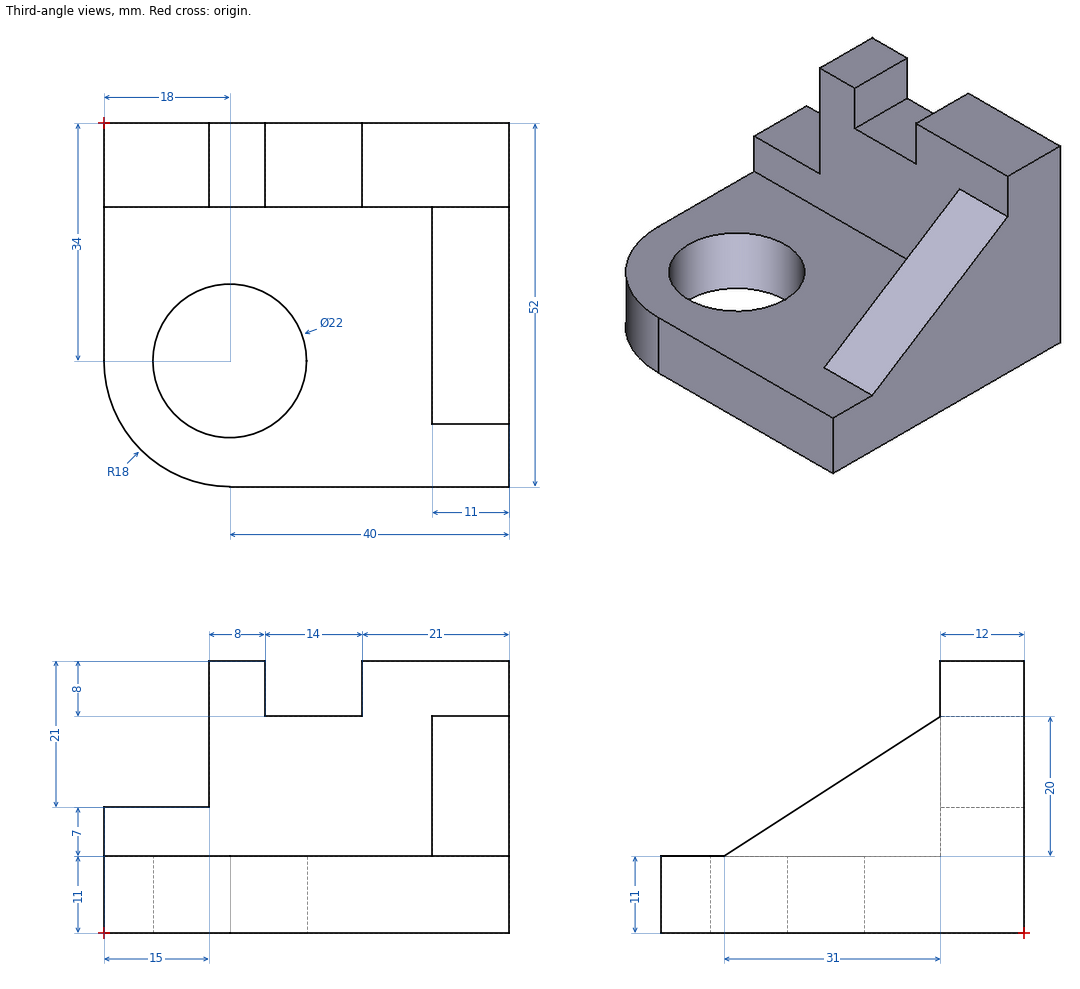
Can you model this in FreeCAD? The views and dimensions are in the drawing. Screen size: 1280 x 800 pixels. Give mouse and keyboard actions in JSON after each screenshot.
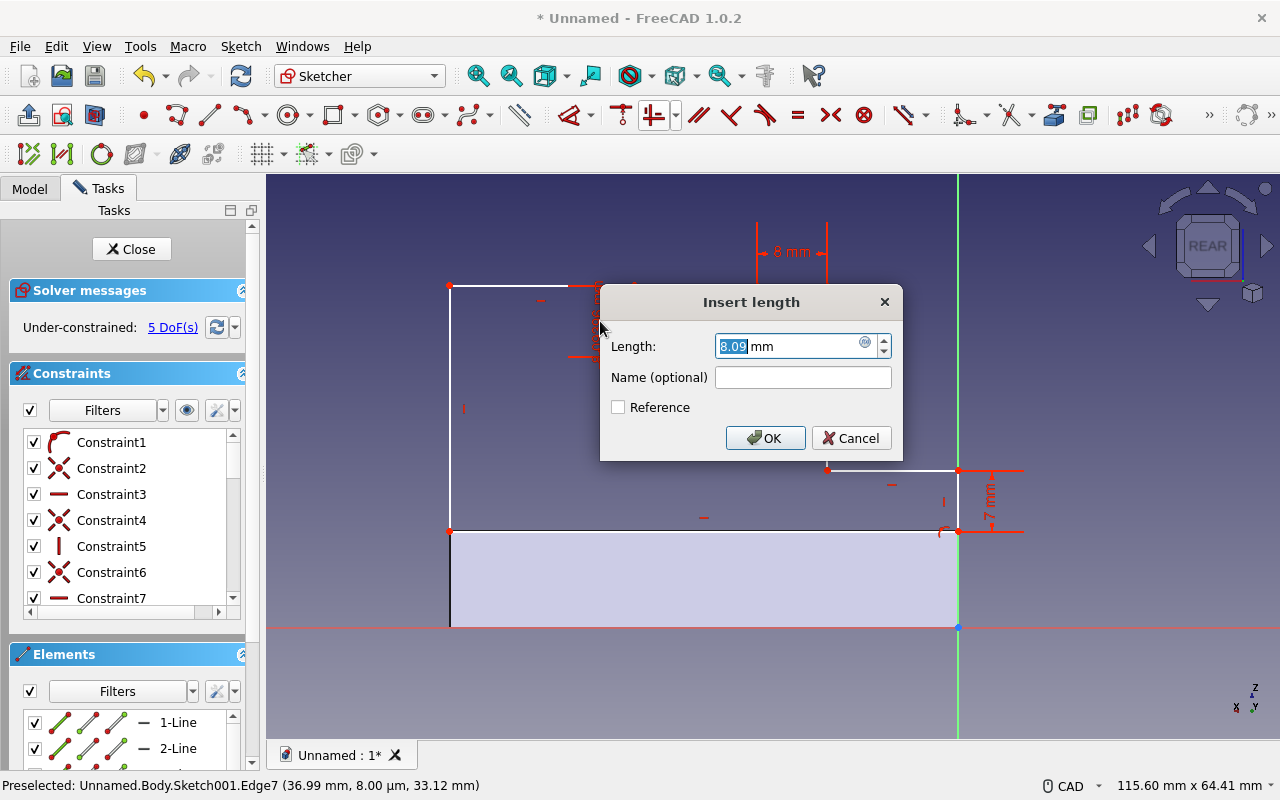
{"action": "type", "text": "8"}
{"action": "key", "text": "Return"}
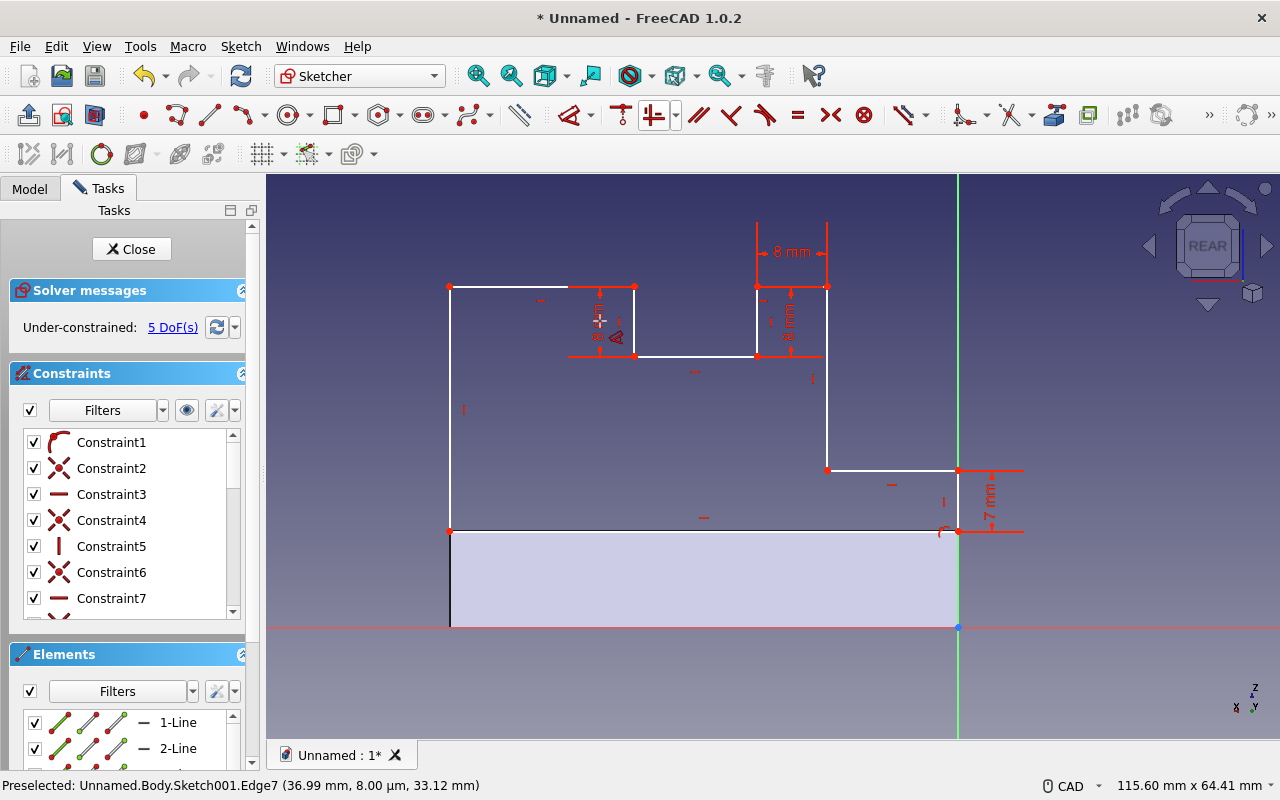
{"action": "left_click", "coordinate": [919, 471]}
{"action": "left_click", "coordinate": [893, 505]}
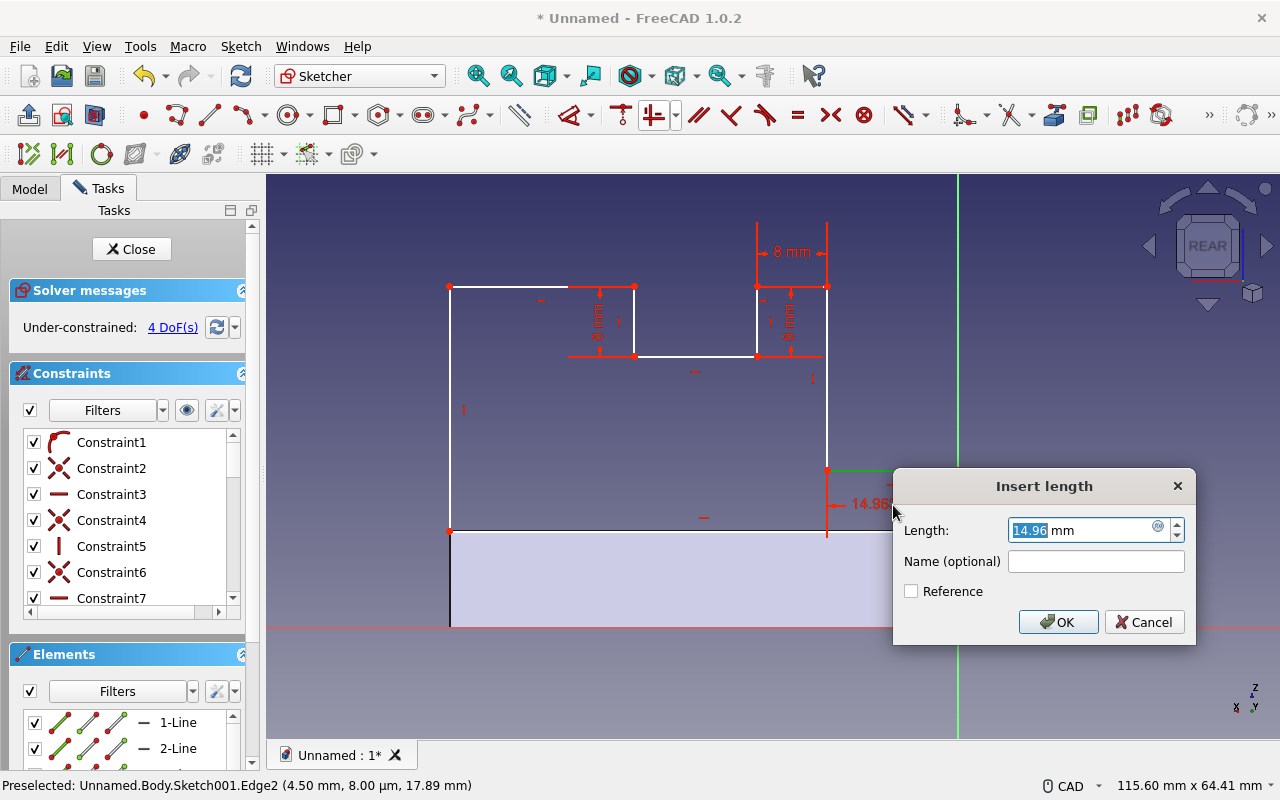
{"action": "type", "text": "15"}
{"action": "key", "text": "Return"}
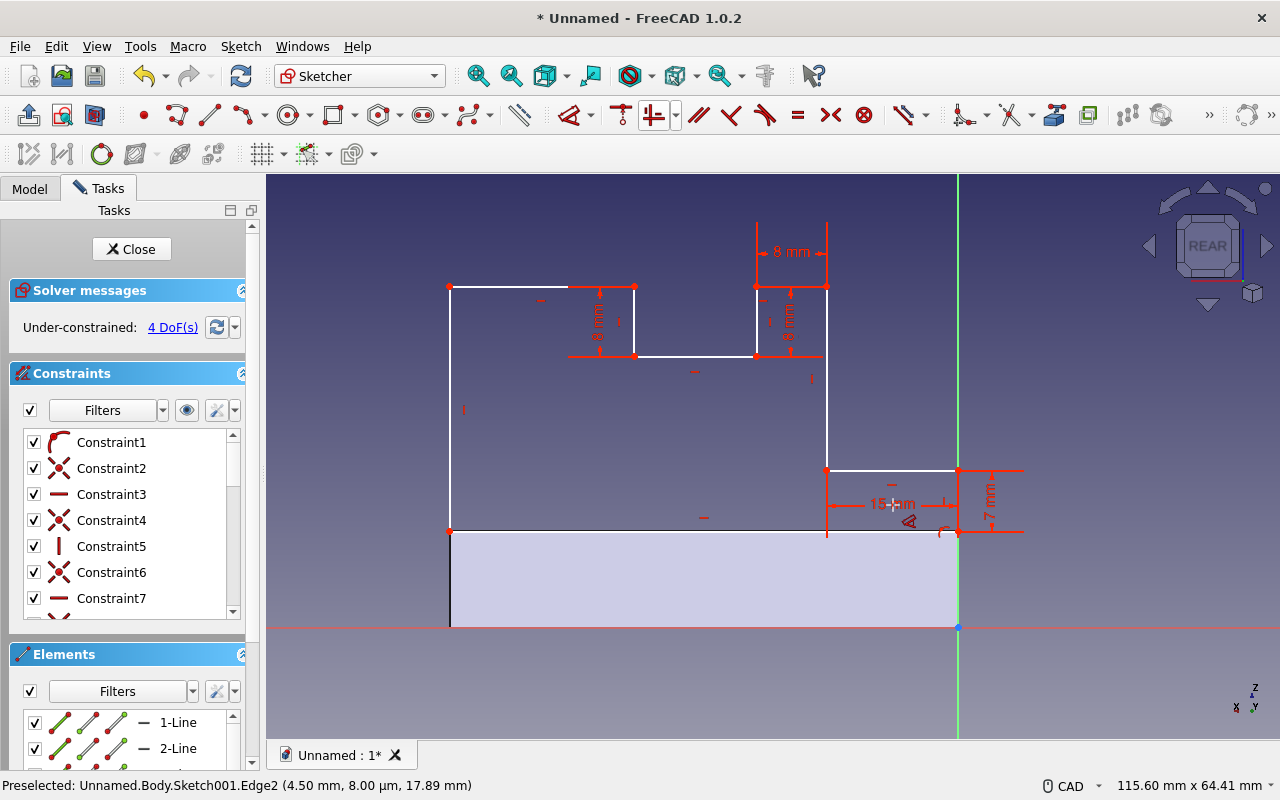
{"action": "left_click", "coordinate": [827, 415]}
{"action": "left_click", "coordinate": [861, 379]}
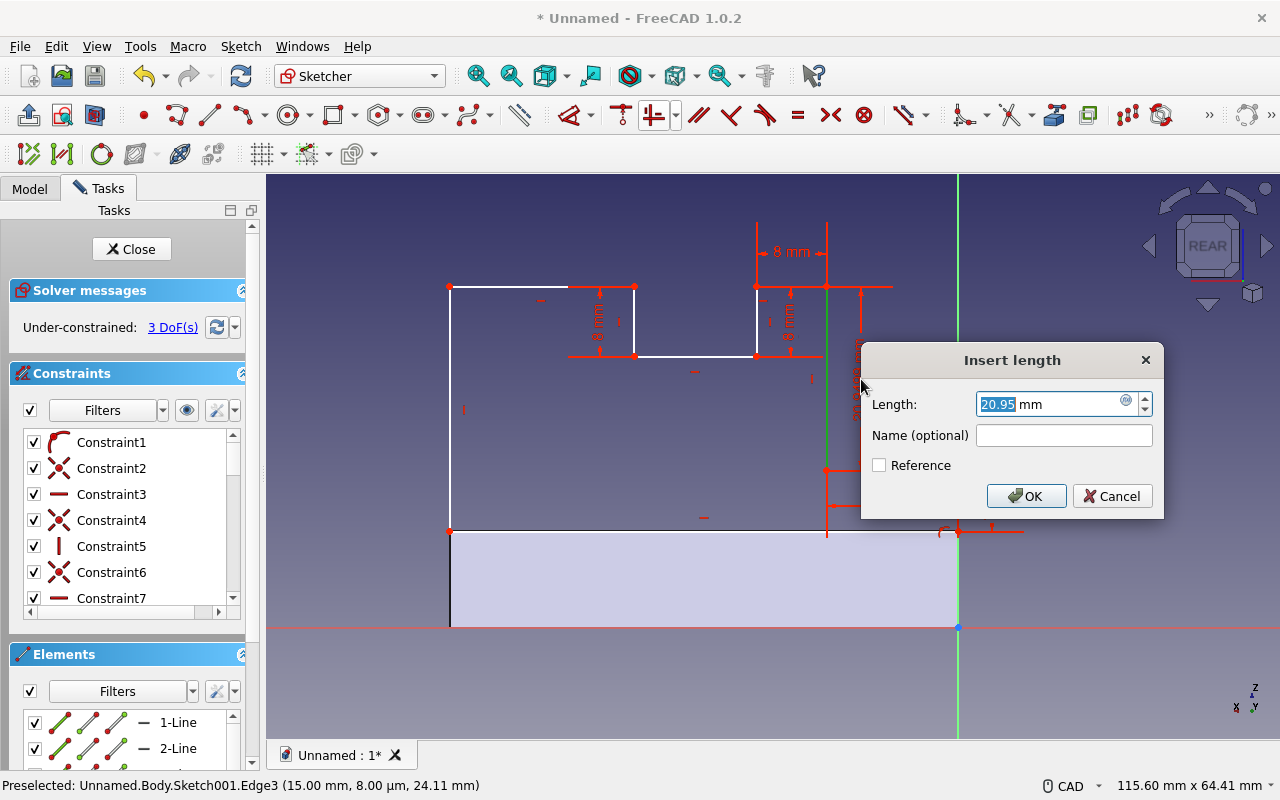
{"action": "type", "text": "21"}
{"action": "key", "text": "Return"}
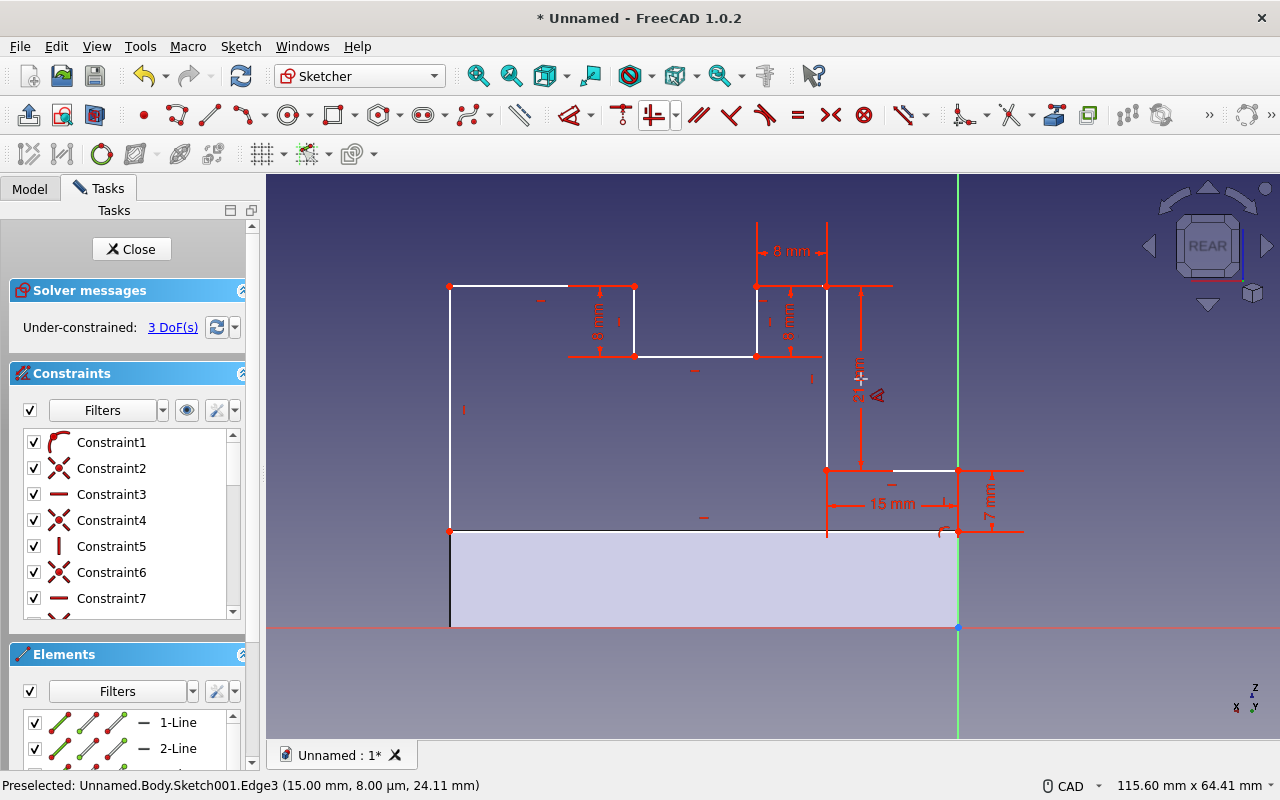
{"action": "left_click", "coordinate": [720, 357]}
{"action": "left_click", "coordinate": [695, 323]}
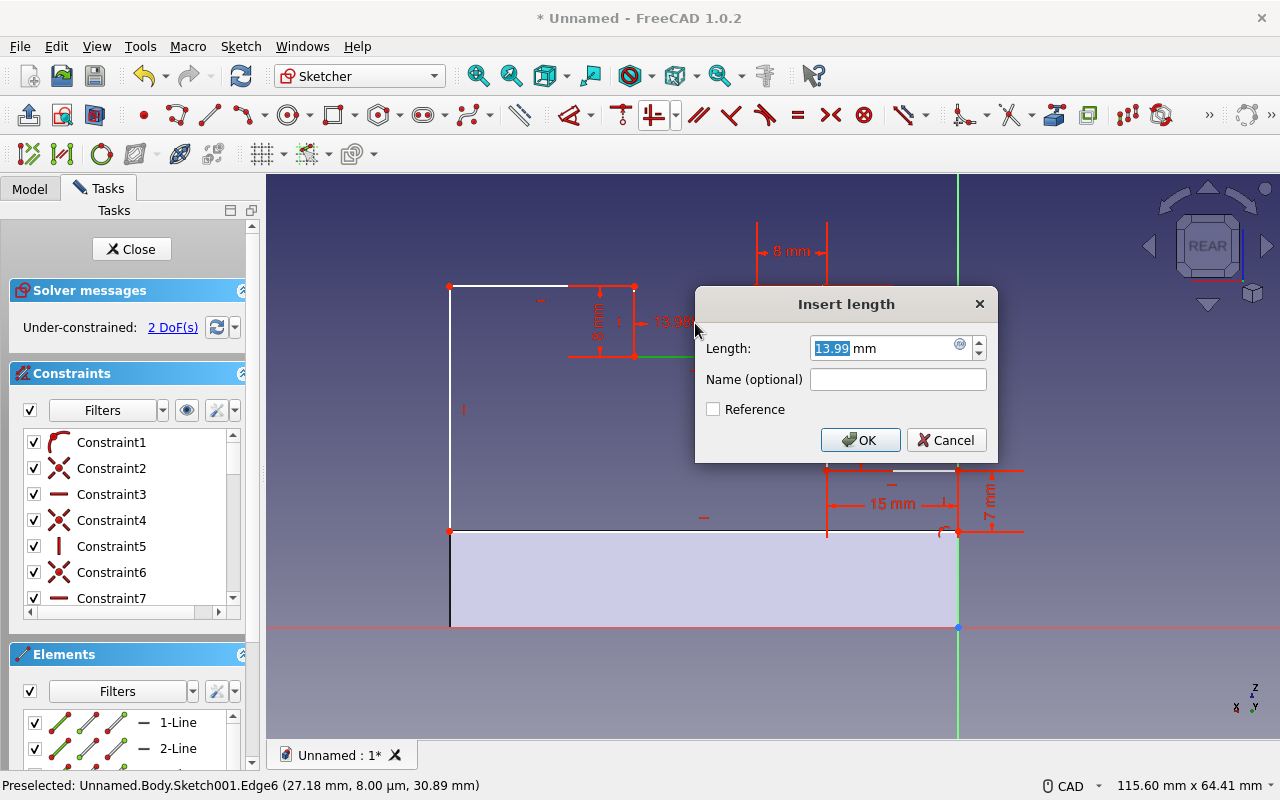
{"action": "type", "text": "14"}
{"action": "key", "text": "Return"}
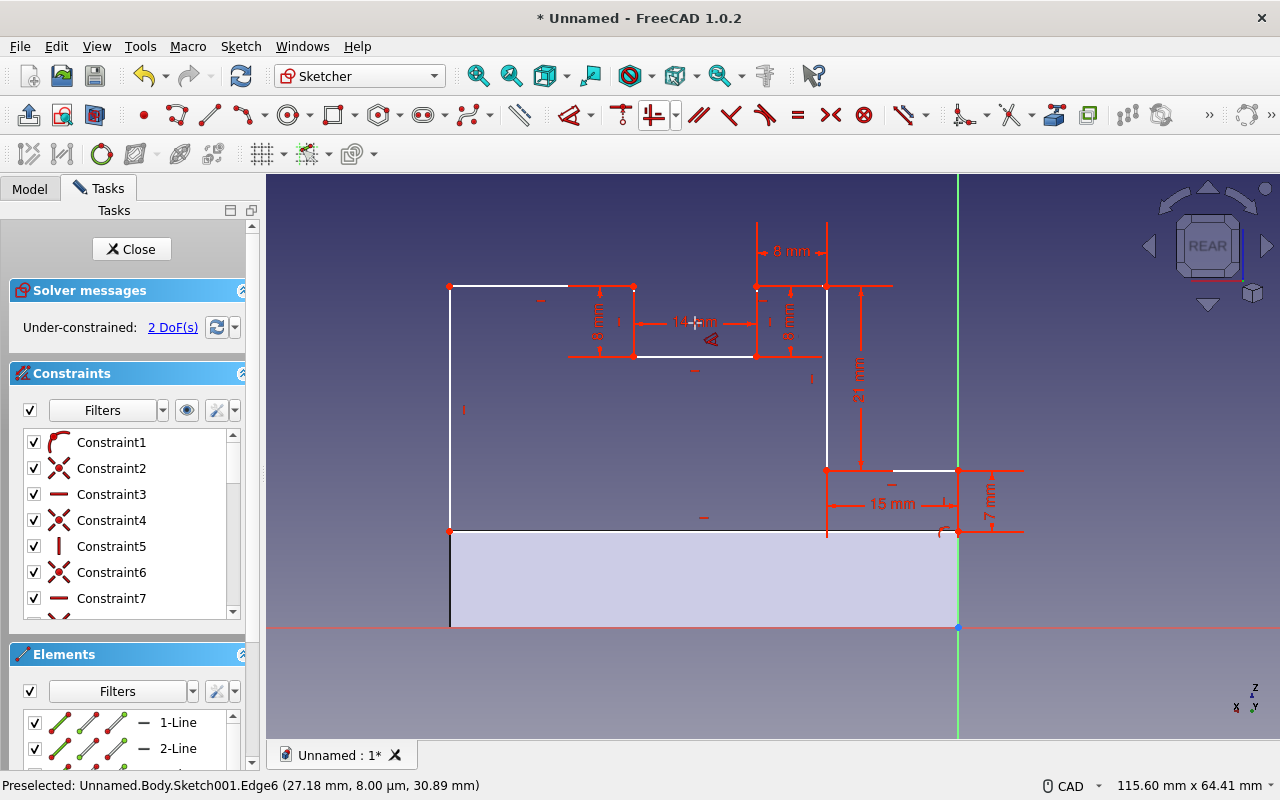
{"action": "left_click", "coordinate": [579, 286]}
{"action": "left_click", "coordinate": [542, 252]}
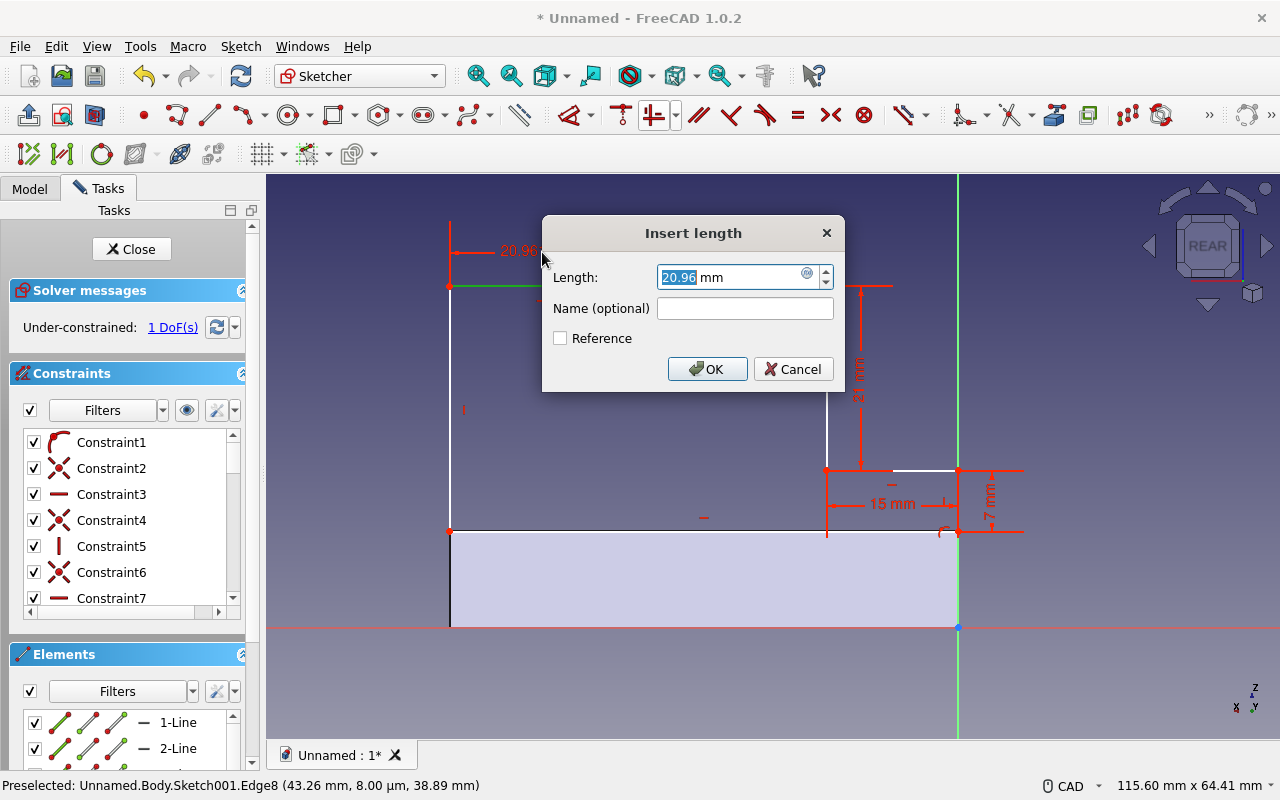
{"action": "type", "text": "21"}
{"action": "key", "text": "Return"}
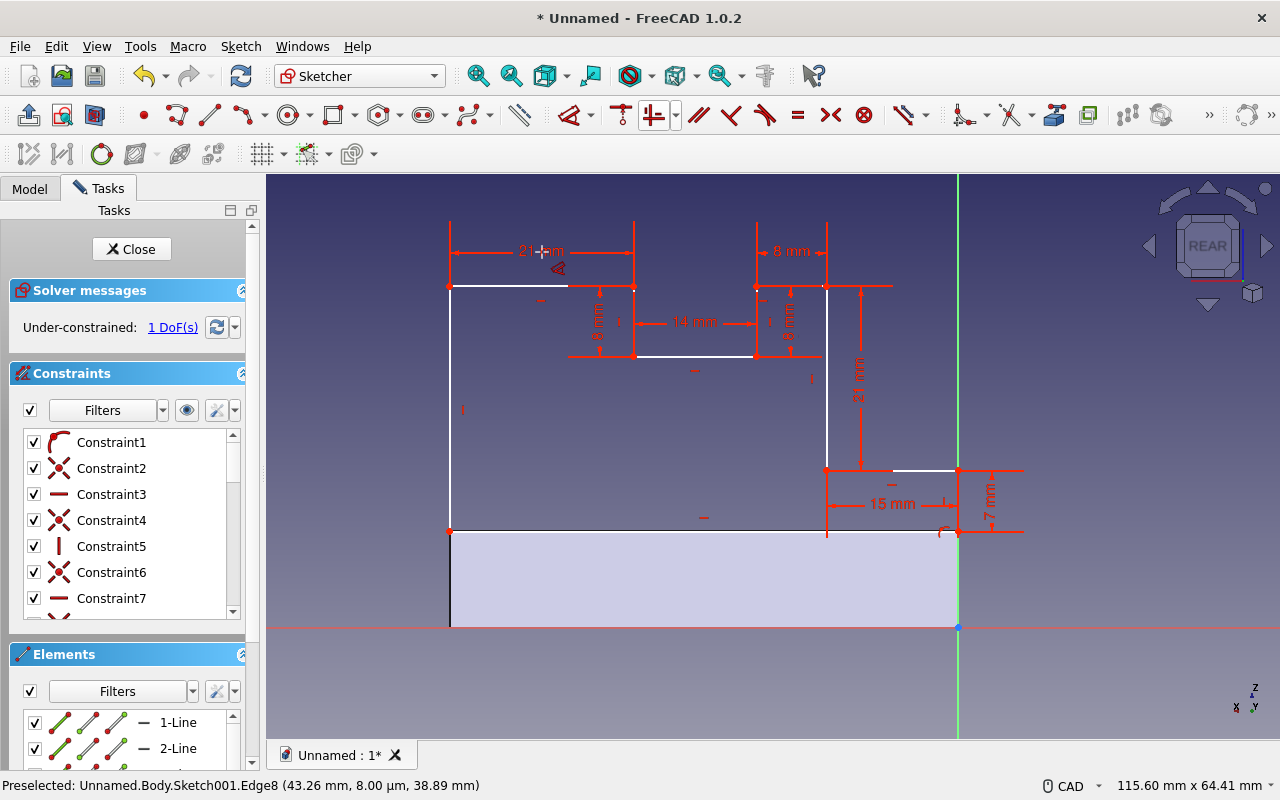
{"action": "left_click", "coordinate": [958, 532]}
{"action": "left_click", "coordinate": [992, 580]}